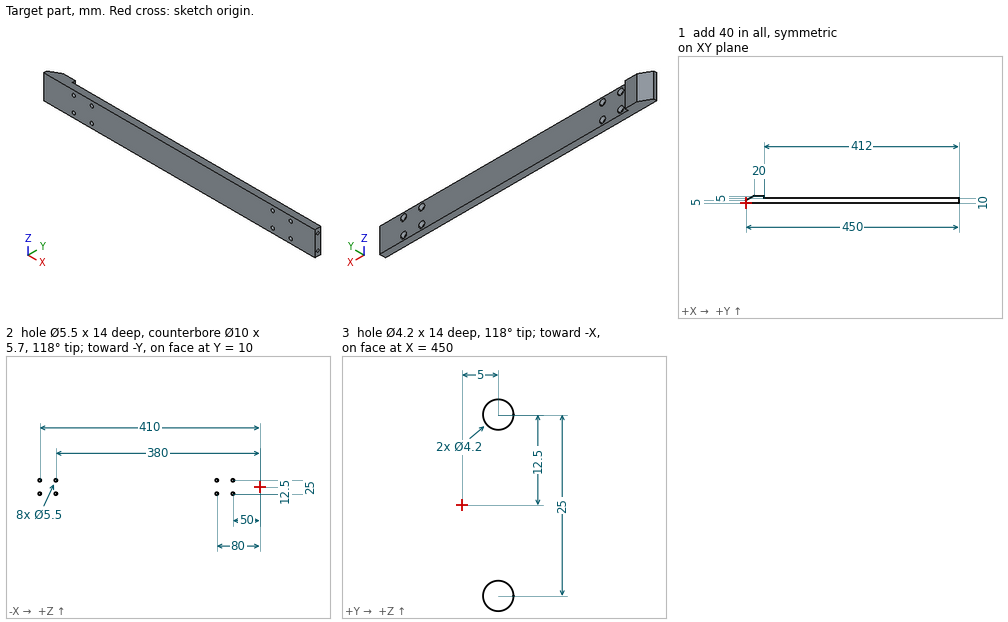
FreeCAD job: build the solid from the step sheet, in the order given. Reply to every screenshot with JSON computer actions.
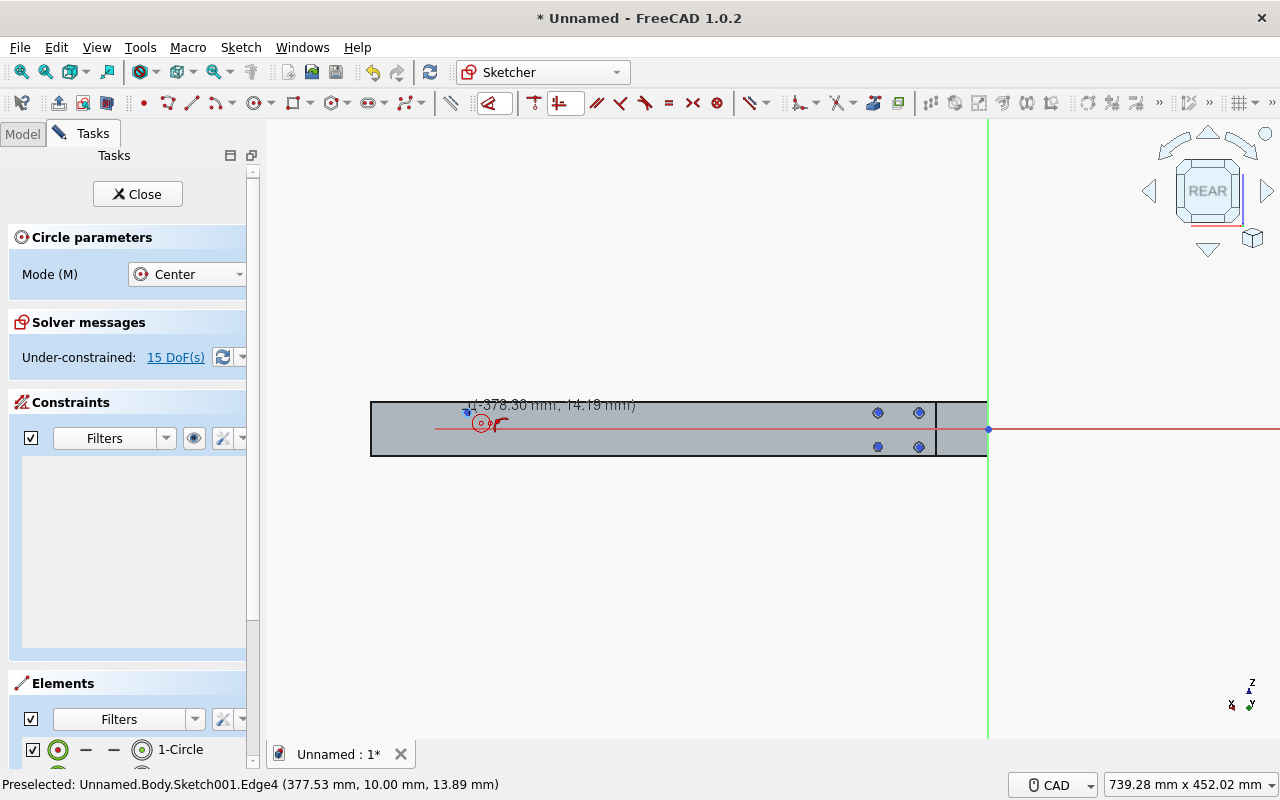
{"action": "scroll", "coordinate": [426, 412], "scroll_direction": "up", "scroll_amount": 9}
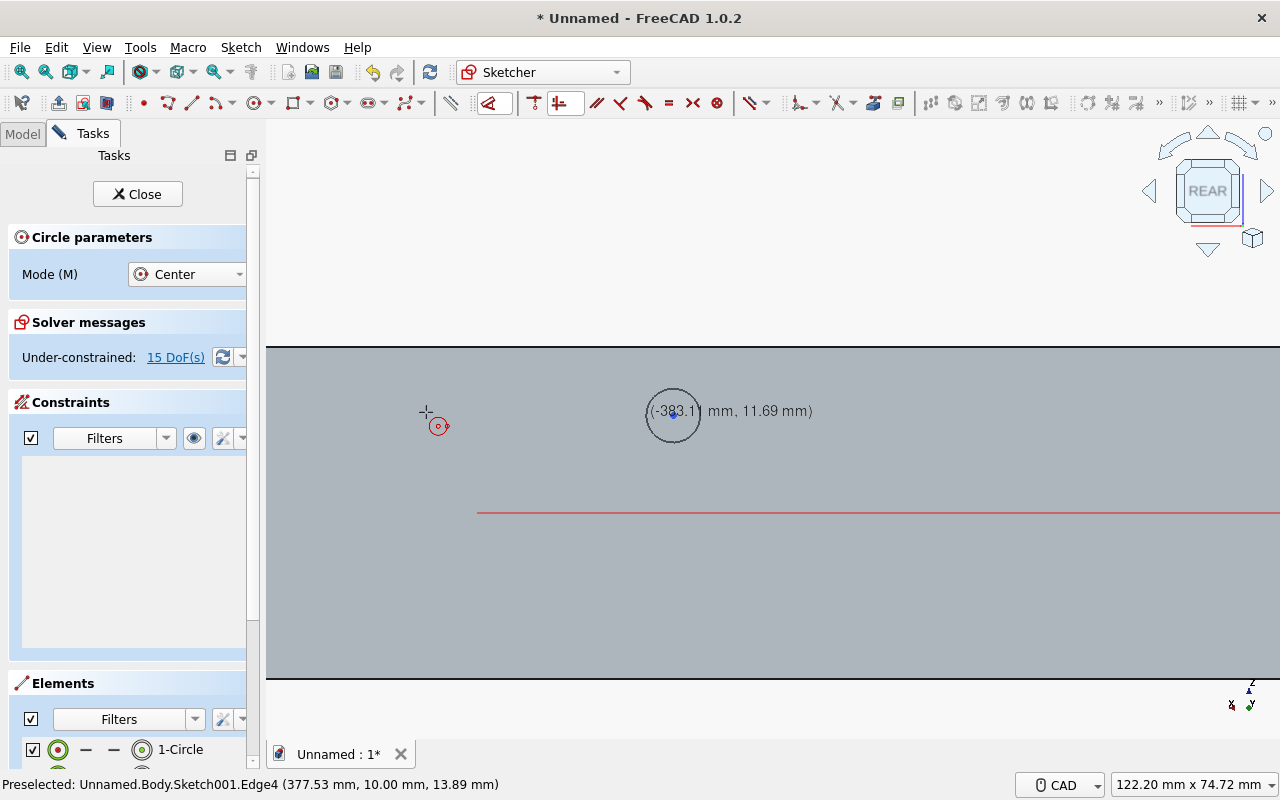
{"action": "scroll", "coordinate": [426, 412], "scroll_direction": "down", "scroll_amount": 9}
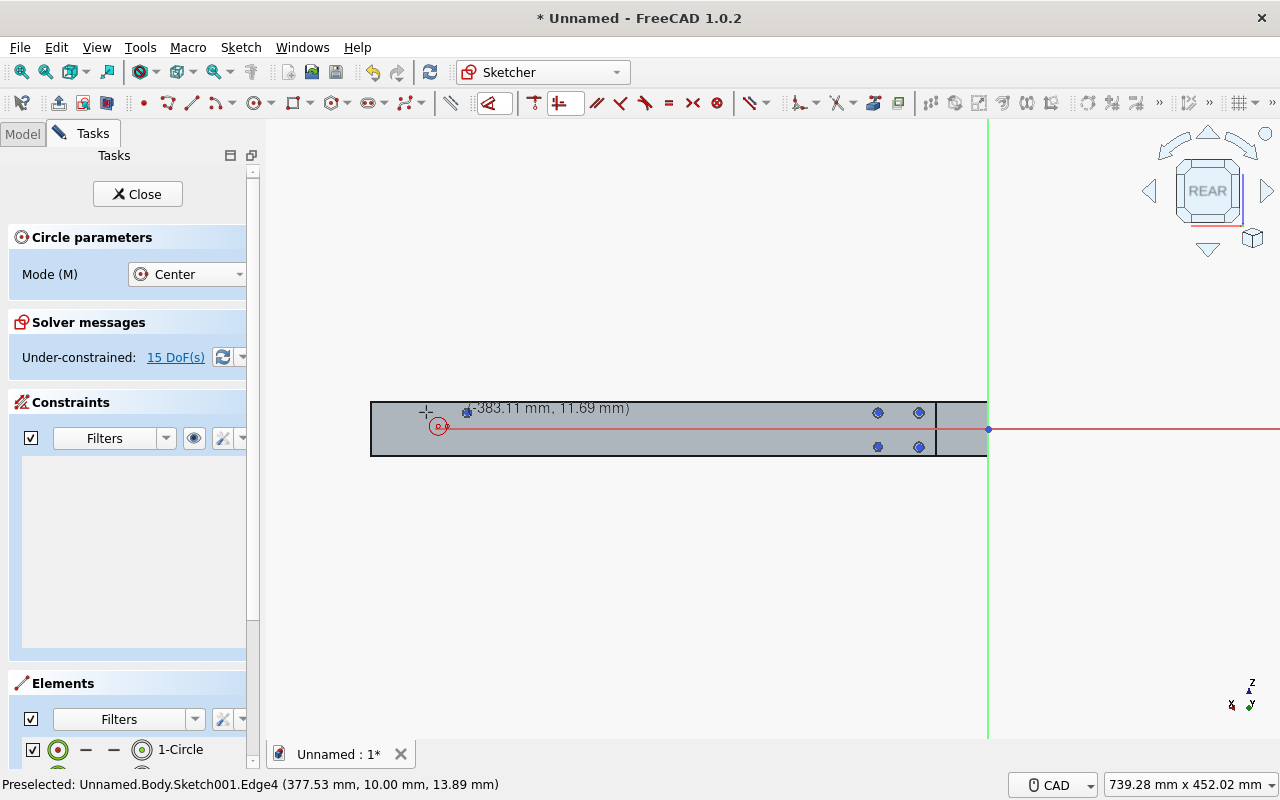
{"action": "left_click", "coordinate": [426, 412]}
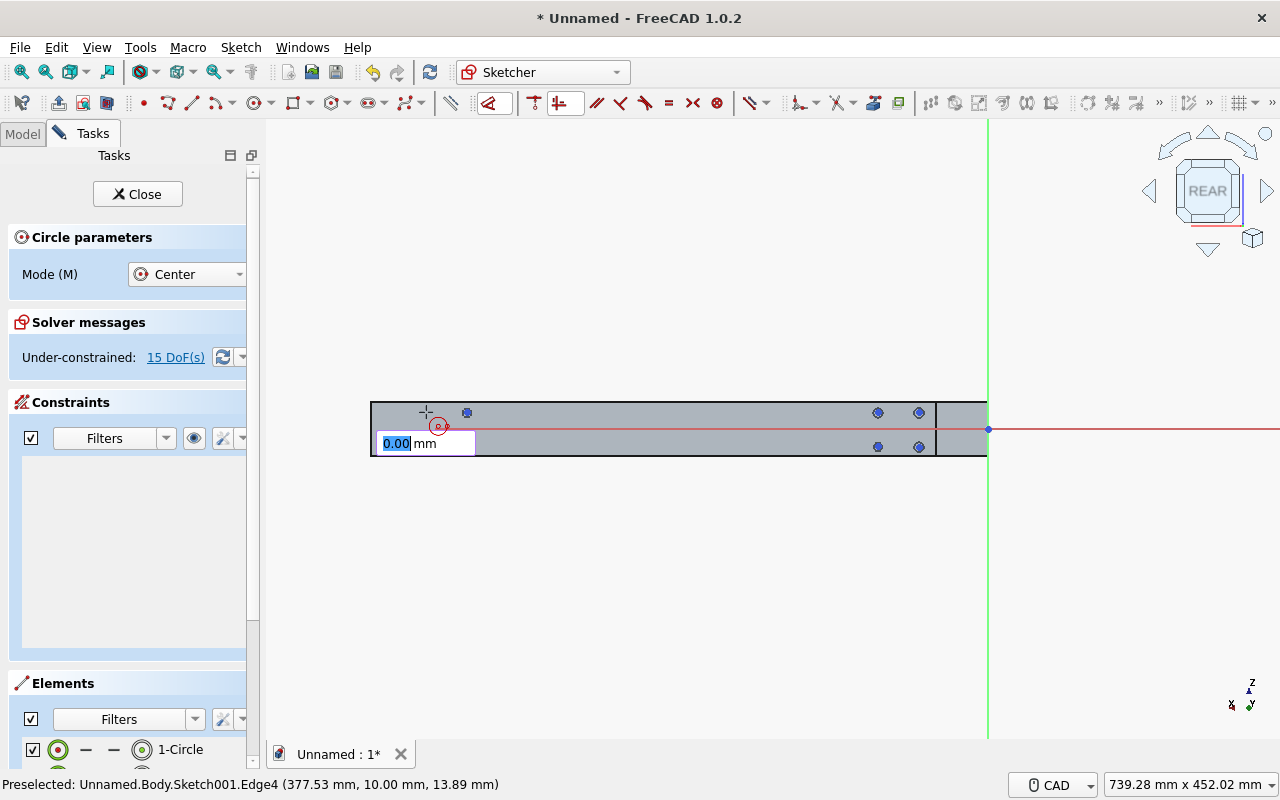
{"action": "scroll", "coordinate": [428, 409], "scroll_direction": "up", "scroll_amount": 8}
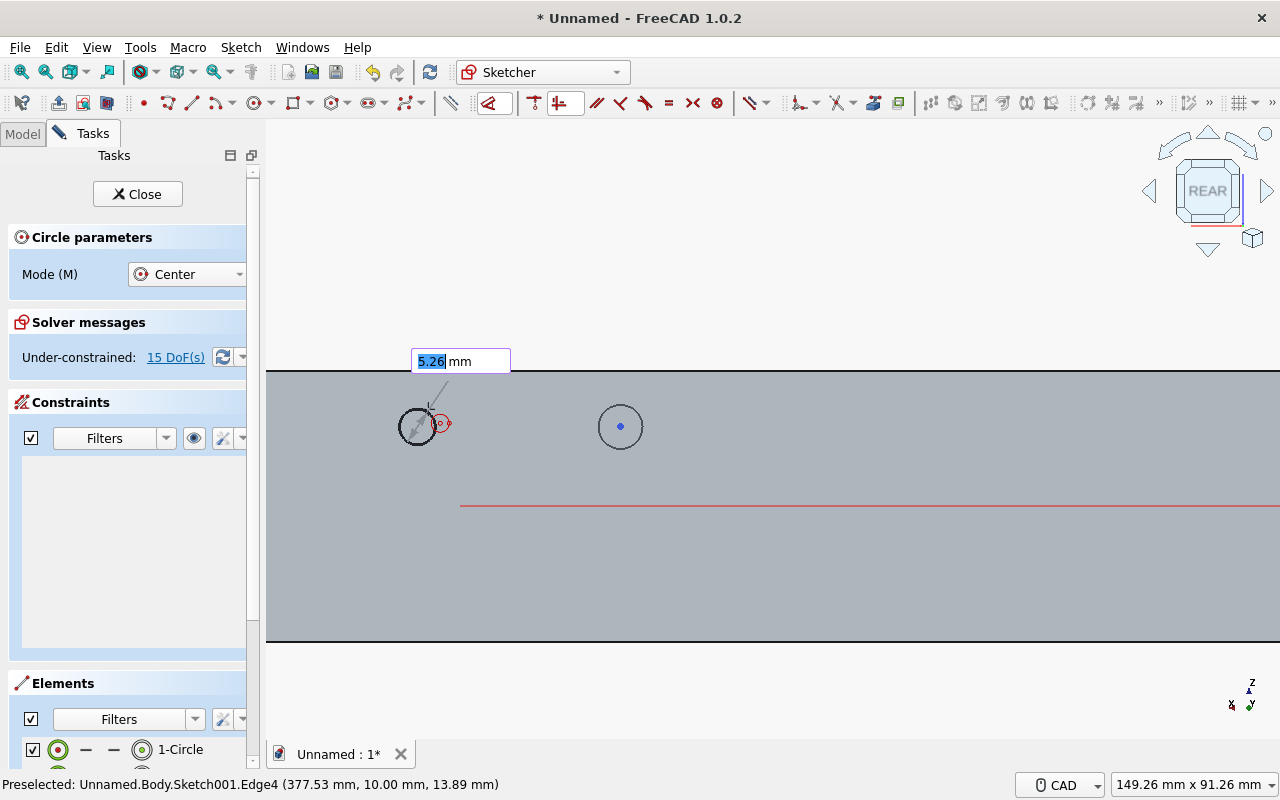
{"action": "left_click", "coordinate": [429, 408]}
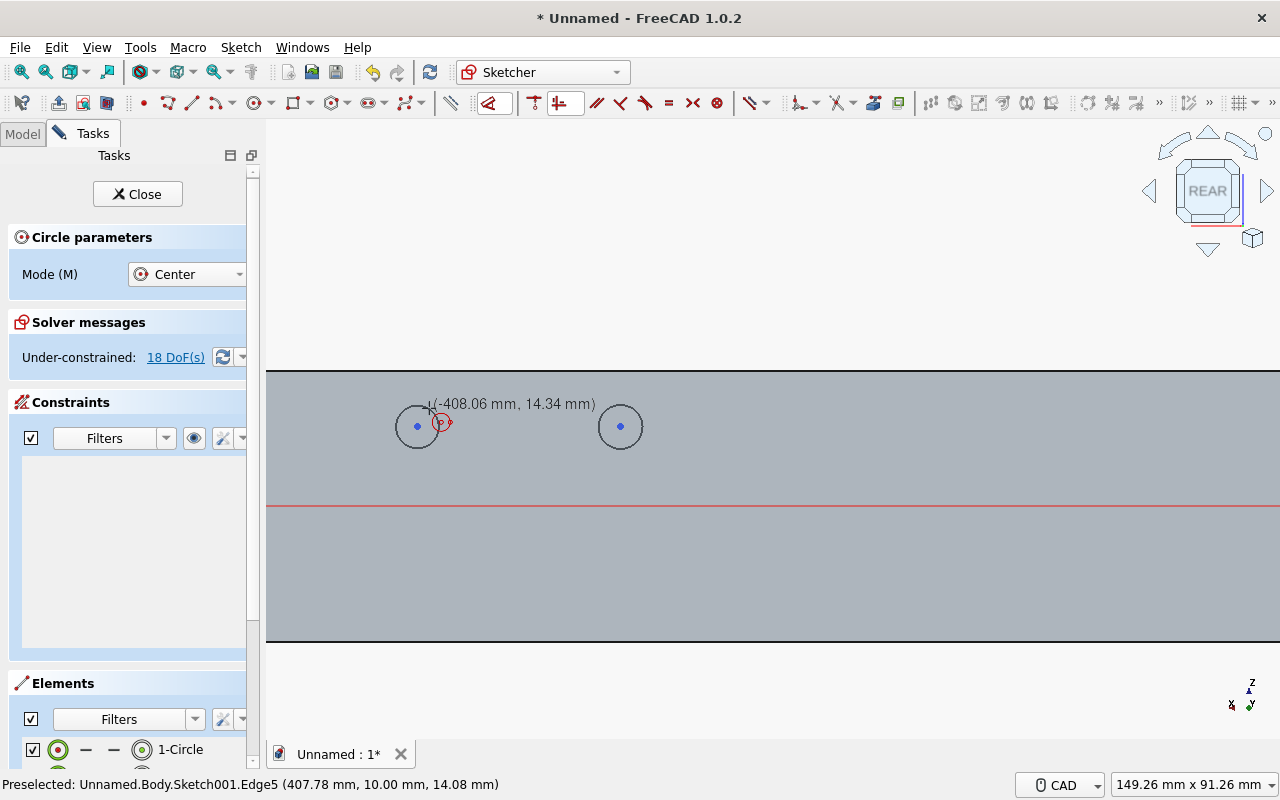
{"action": "scroll", "coordinate": [428, 409], "scroll_direction": "down", "scroll_amount": 8}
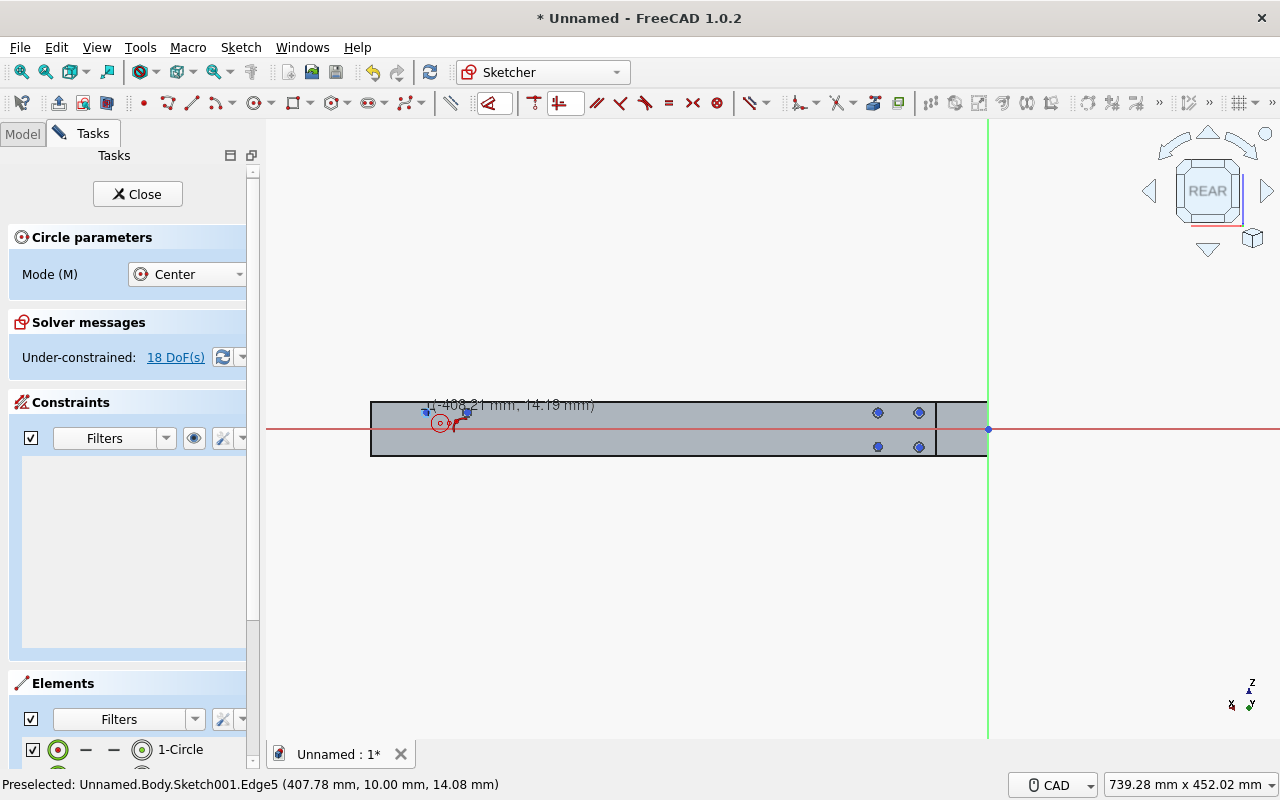
{"action": "left_click", "coordinate": [467, 446]}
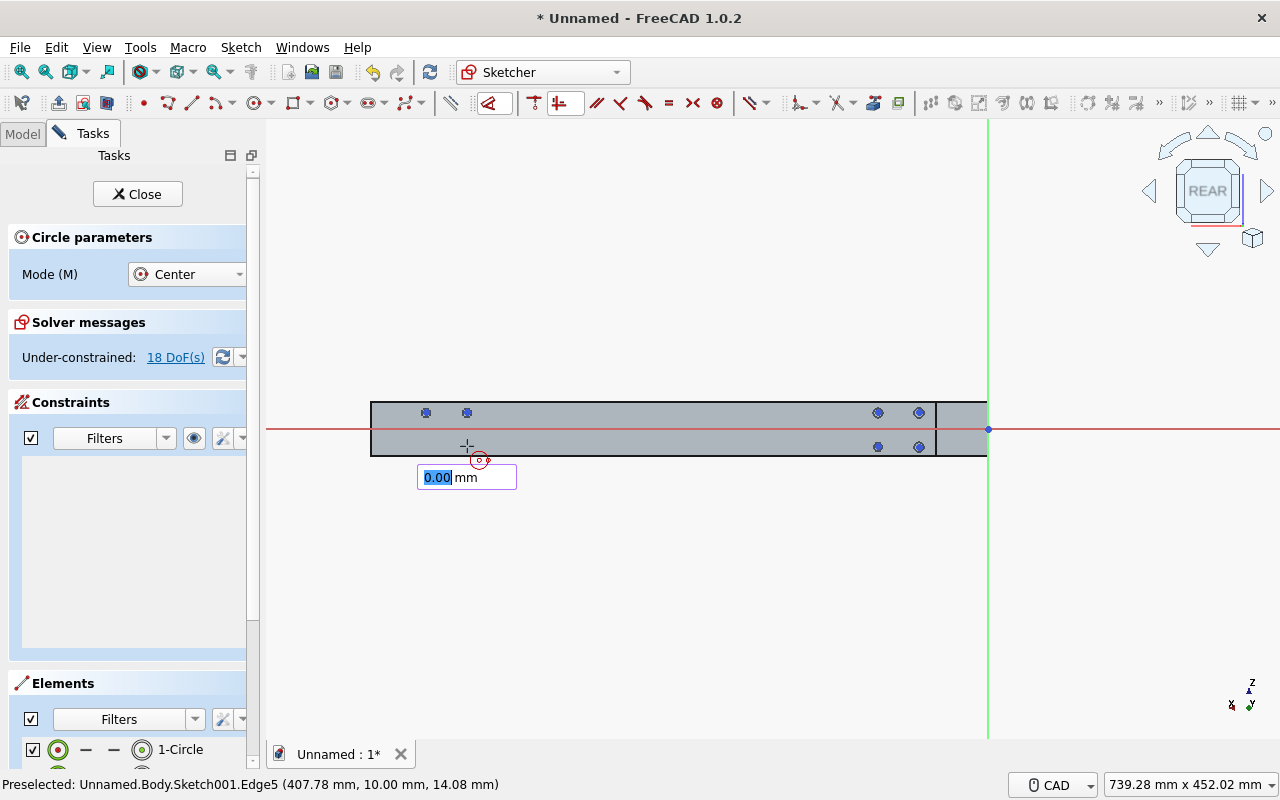
{"action": "scroll", "coordinate": [469, 444], "scroll_direction": "up", "scroll_amount": 8}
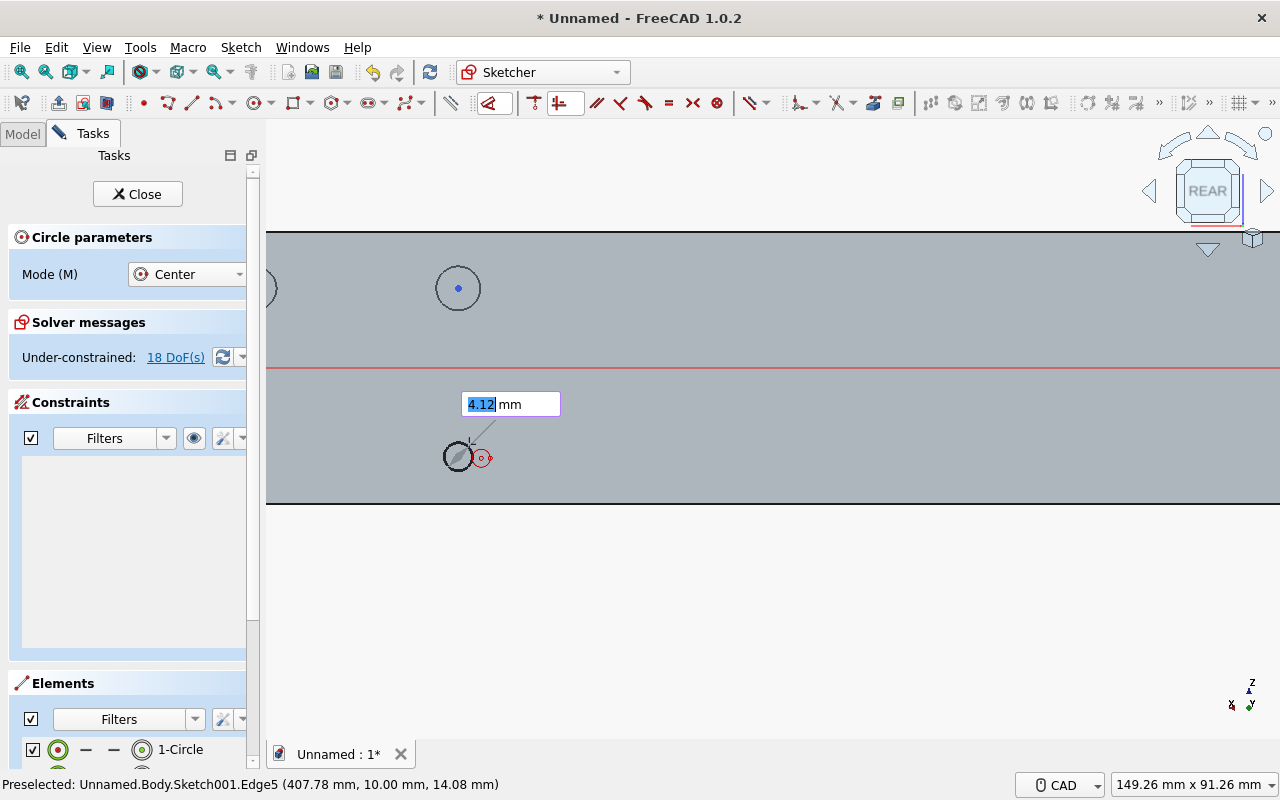
{"action": "left_click", "coordinate": [471, 440]}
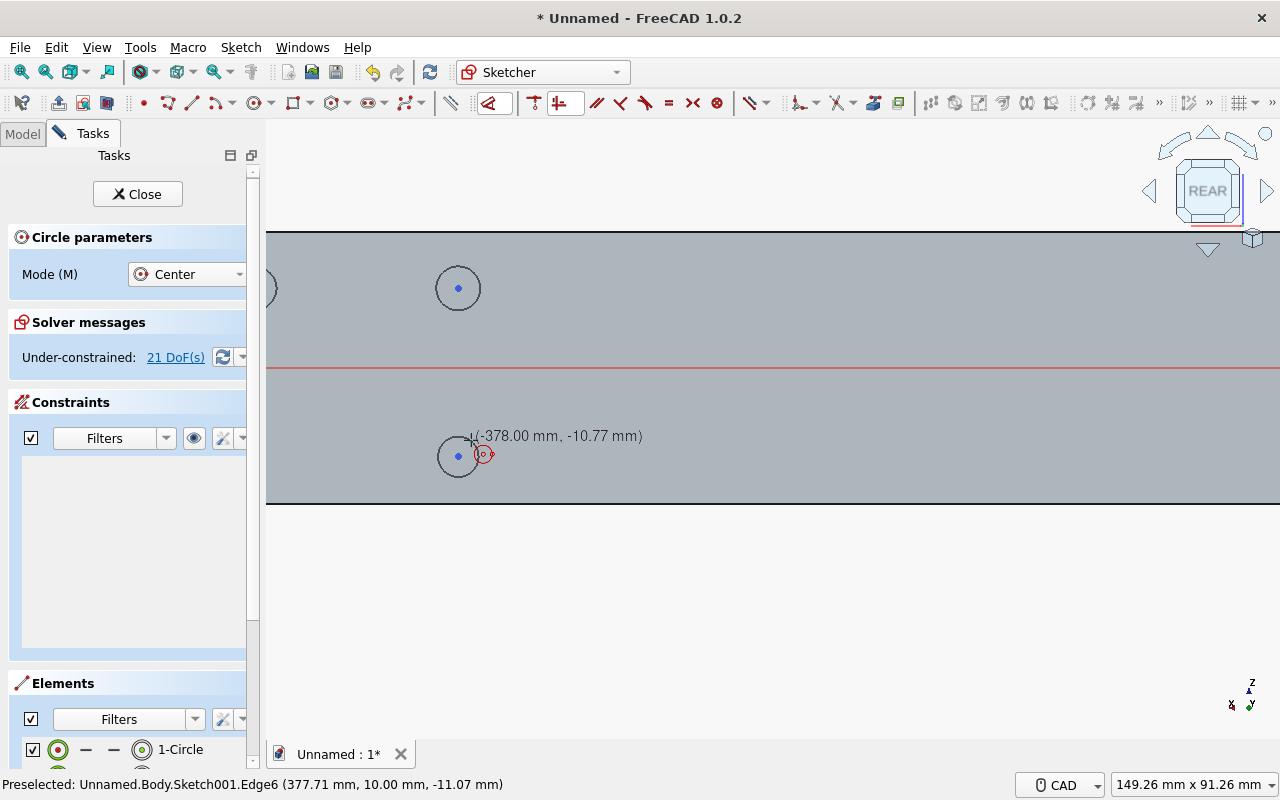
{"action": "scroll", "coordinate": [469, 444], "scroll_direction": "down", "scroll_amount": 8}